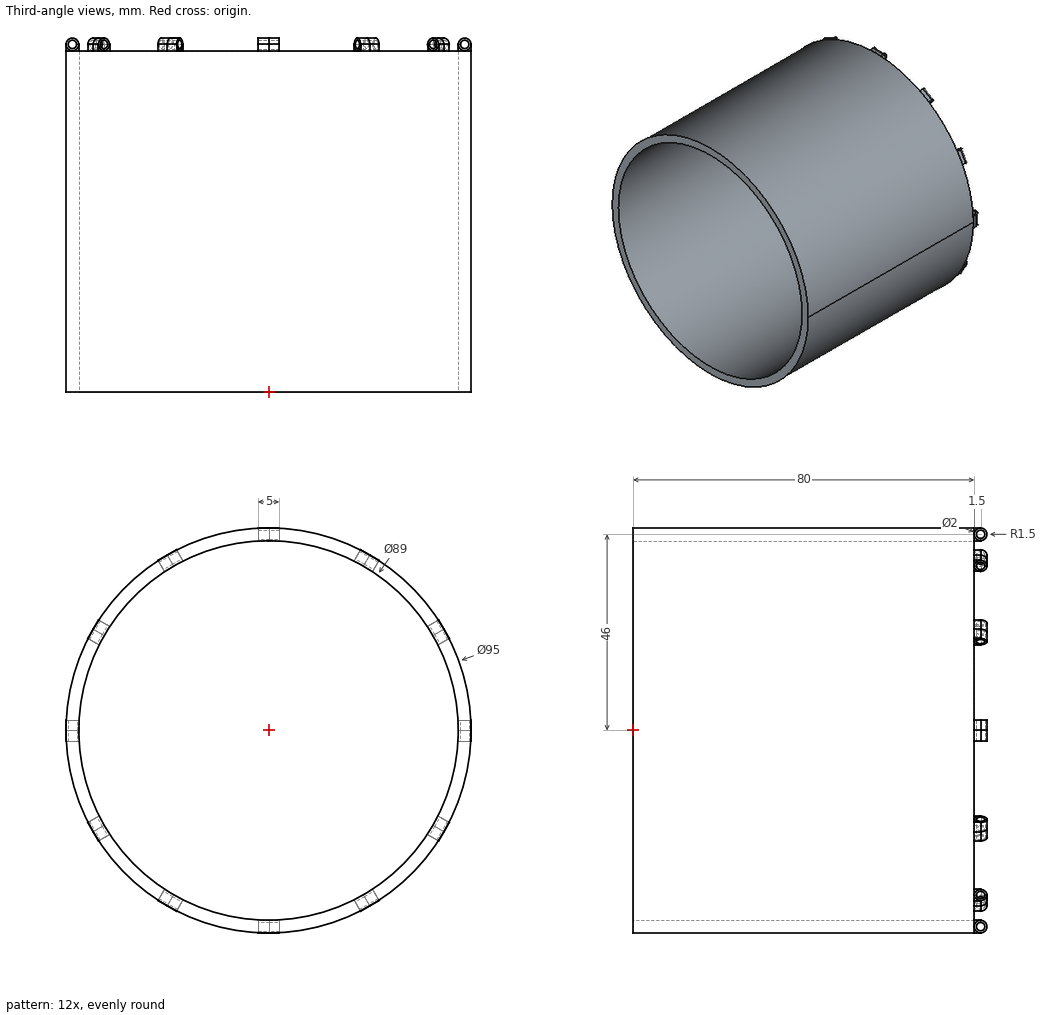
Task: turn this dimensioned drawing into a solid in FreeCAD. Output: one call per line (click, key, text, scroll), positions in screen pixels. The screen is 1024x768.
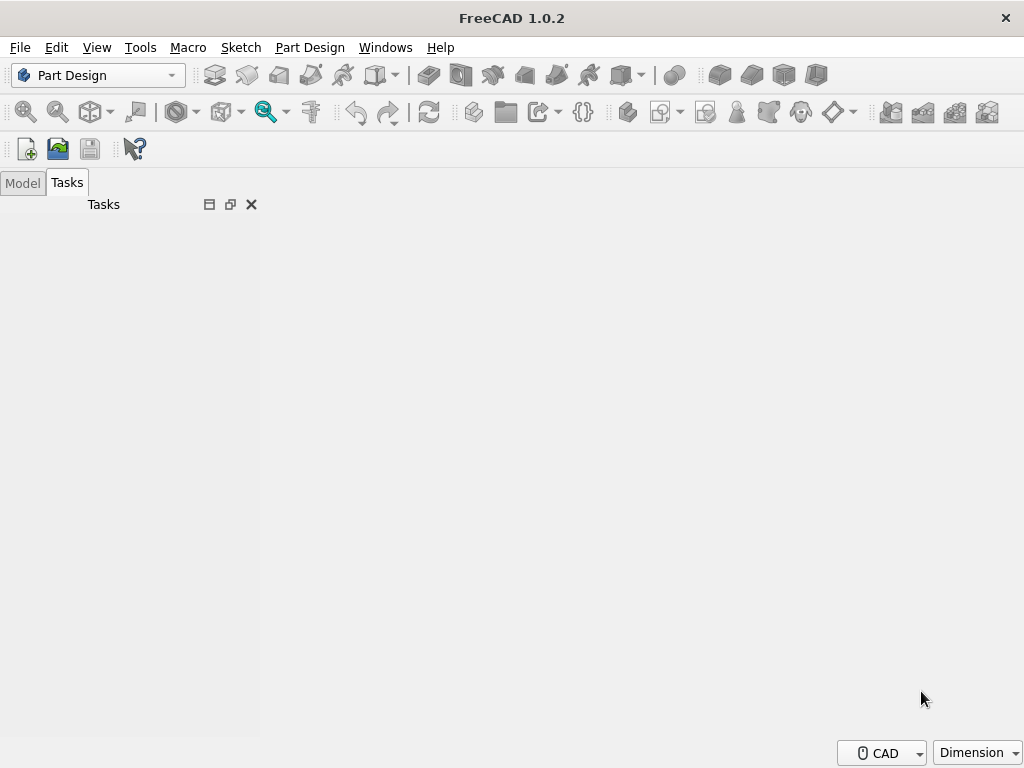
click(26, 150)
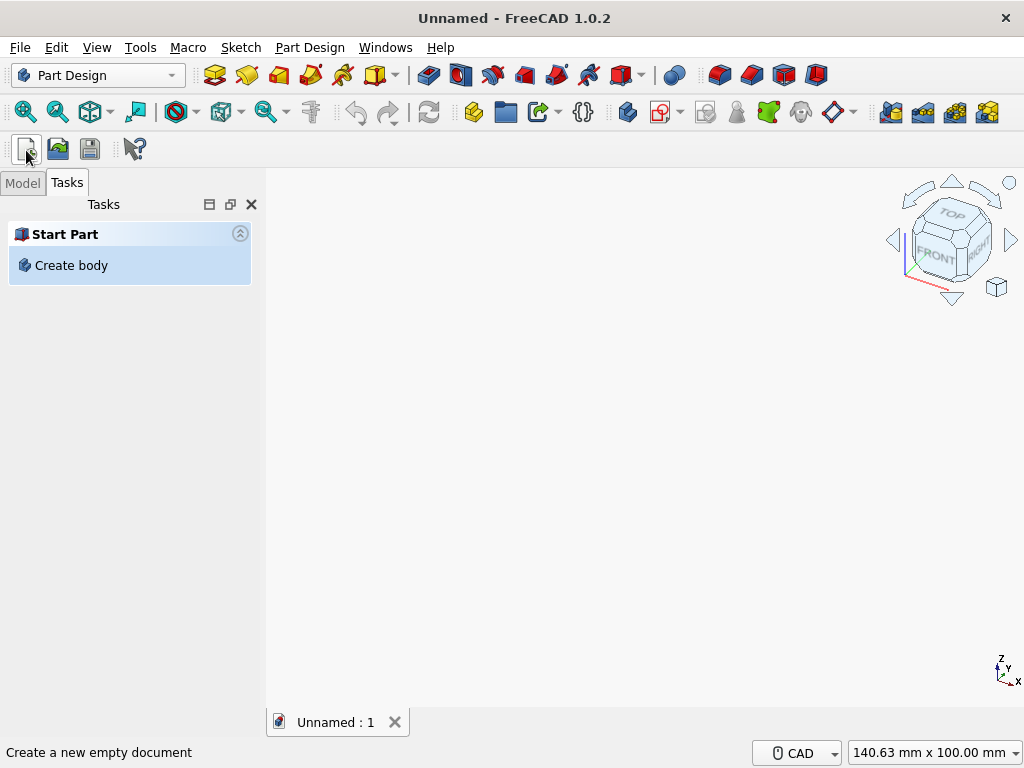
click(660, 112)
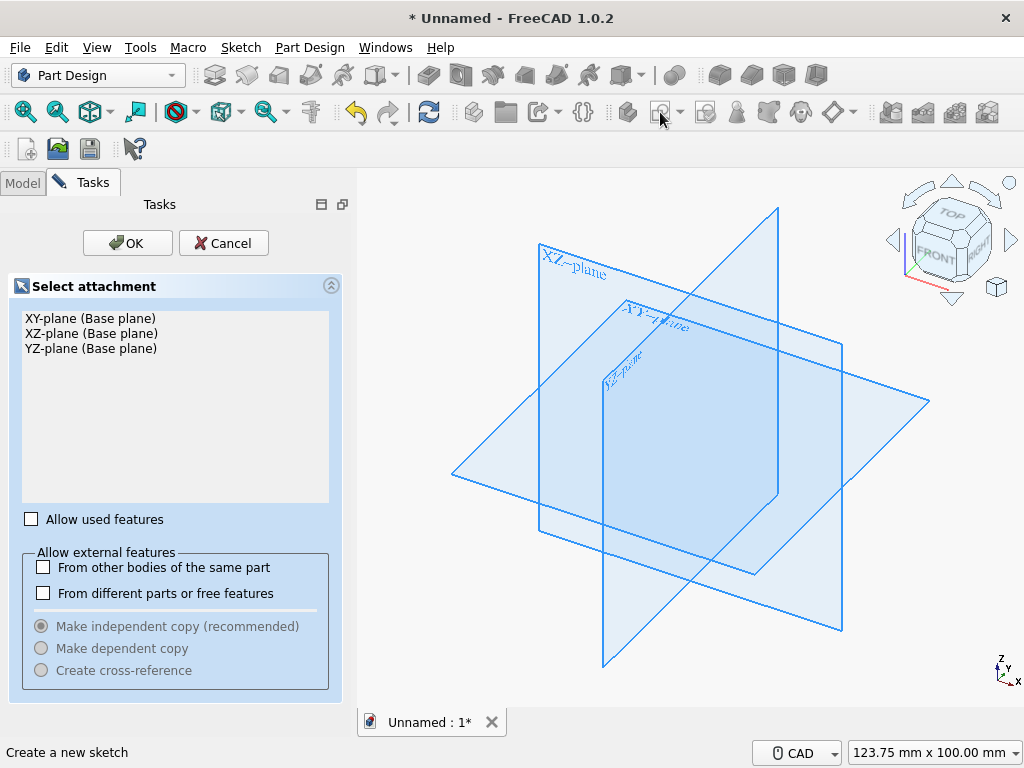
click(82, 334)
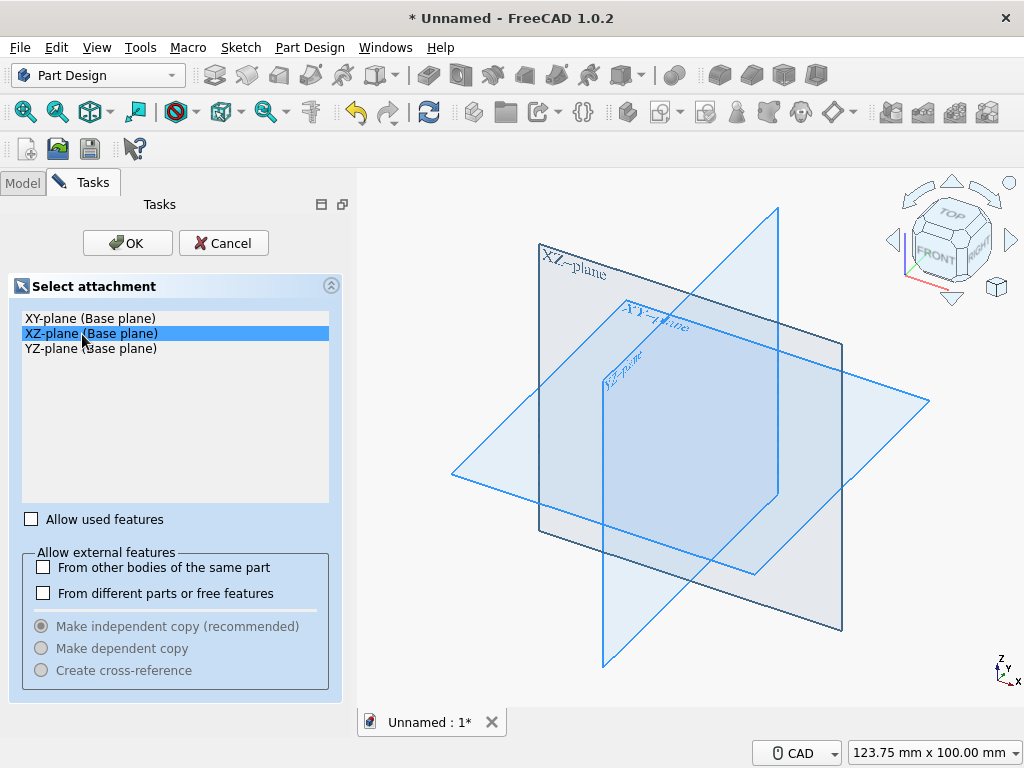
click(128, 243)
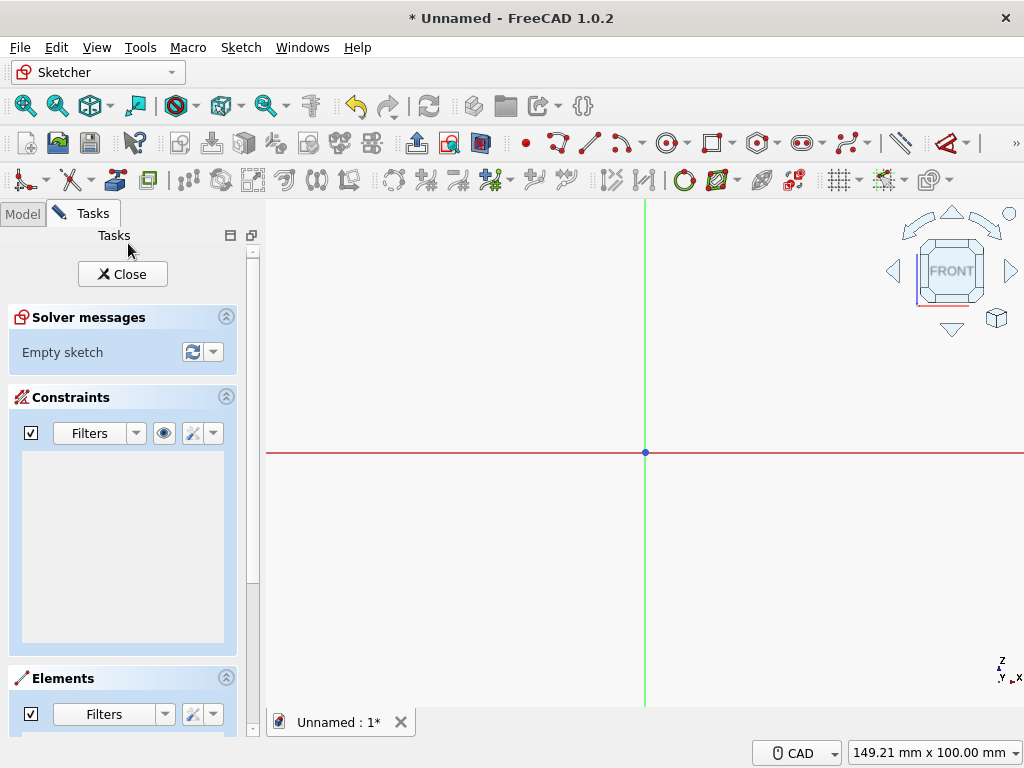
scroll(437, 453, down, 2)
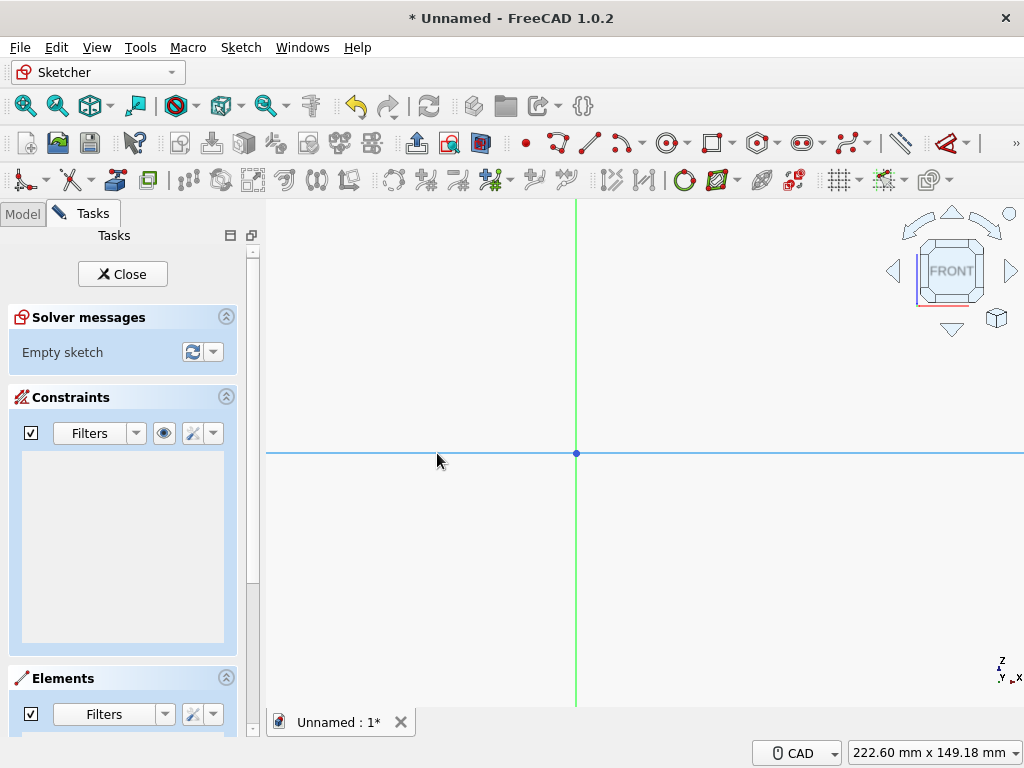
click(668, 144)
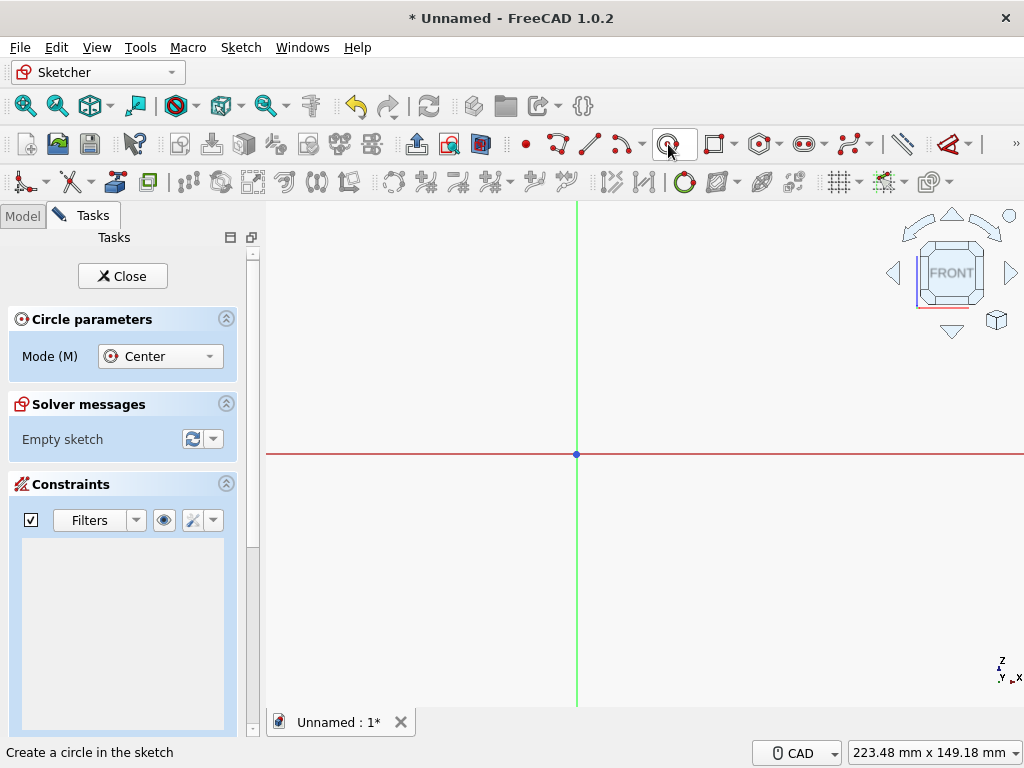
click(577, 454)
click(691, 340)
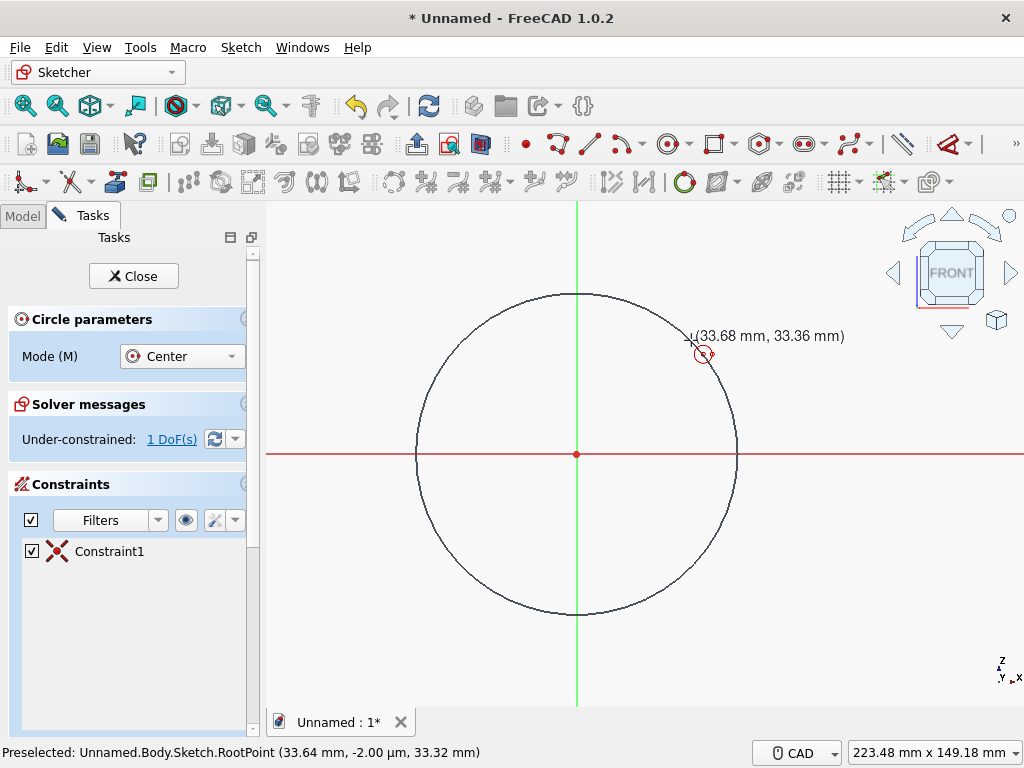
click(577, 454)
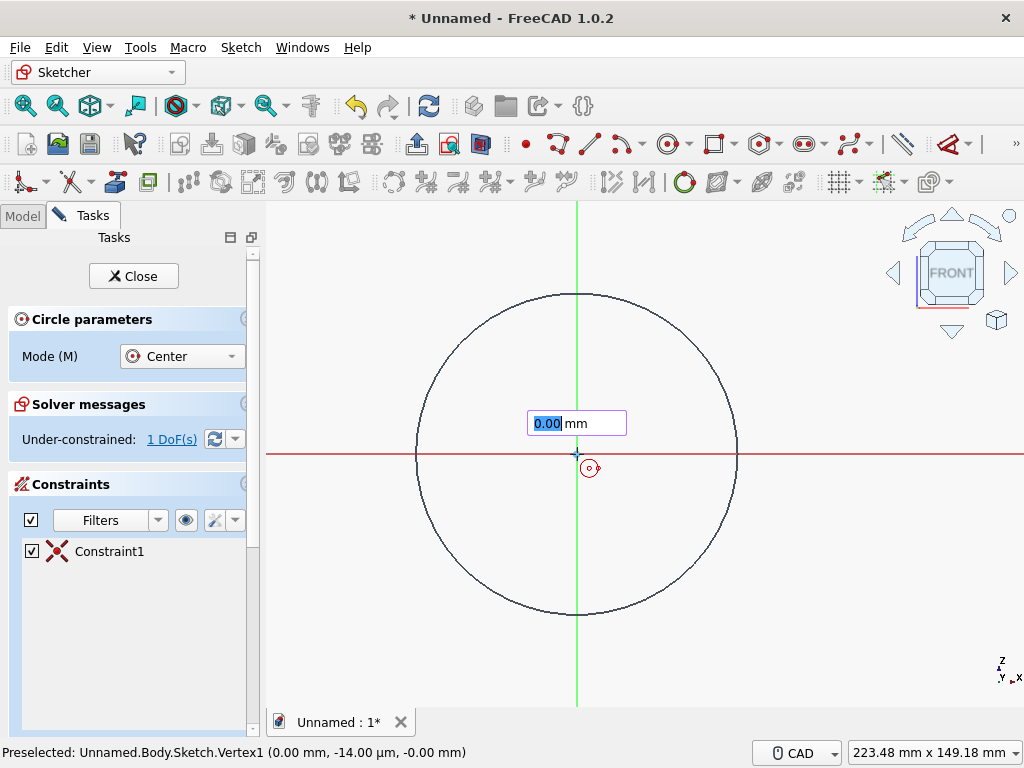
scroll(525, 596, up, 3)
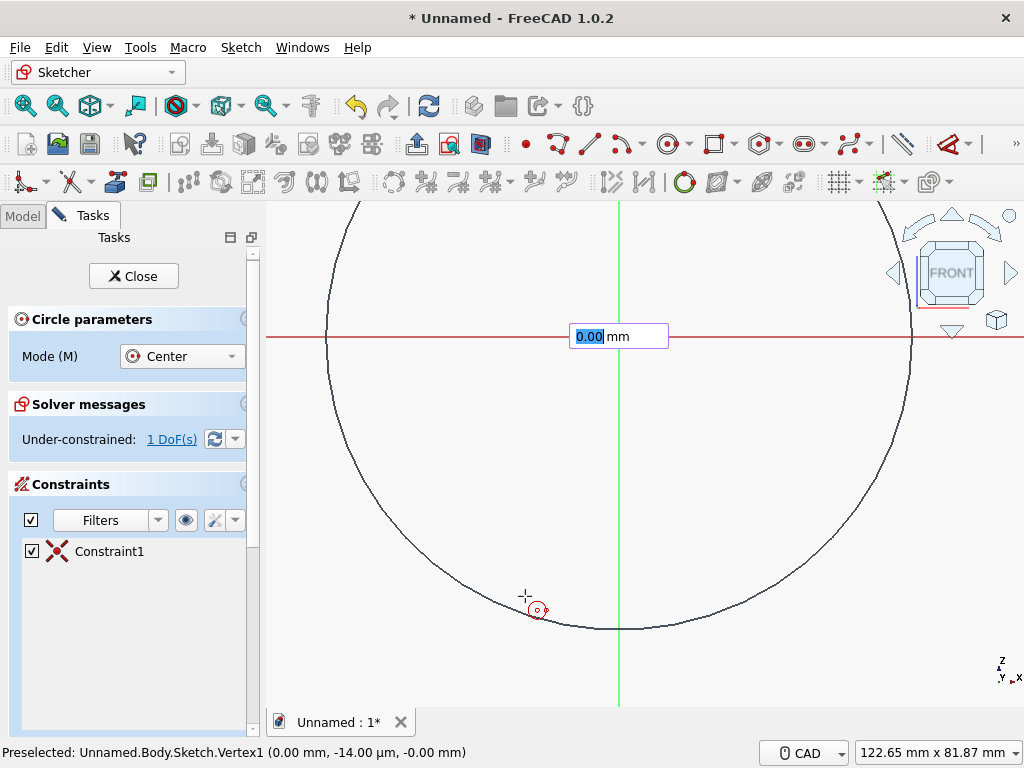
click(525, 595)
key(Escape)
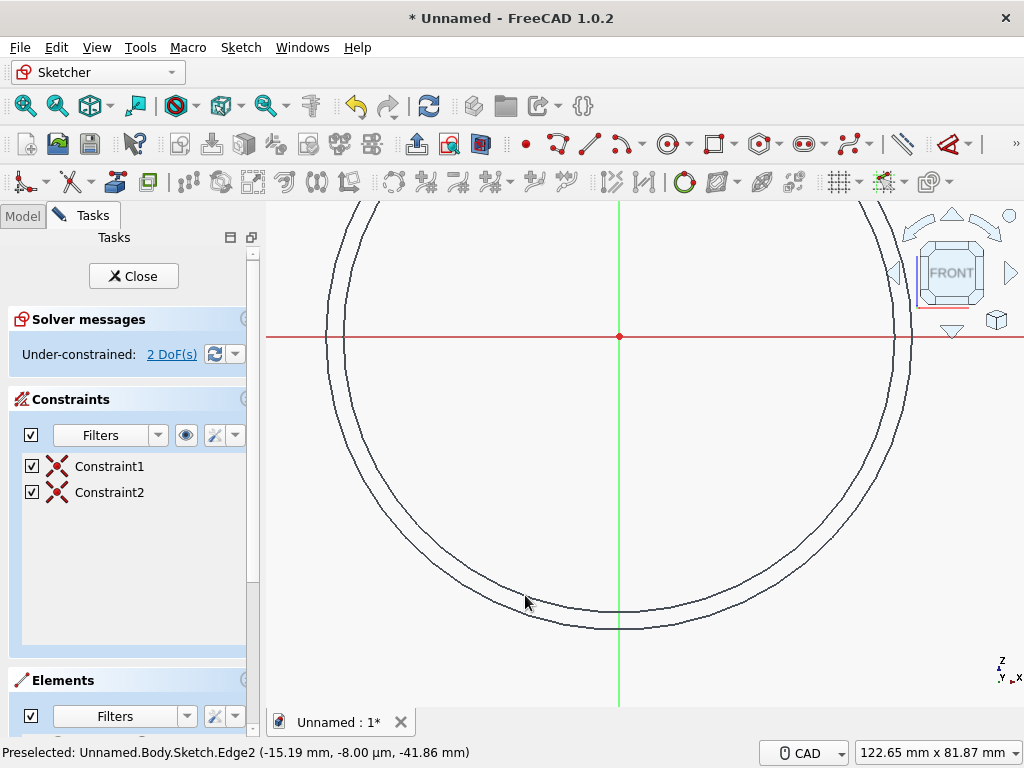
click(948, 144)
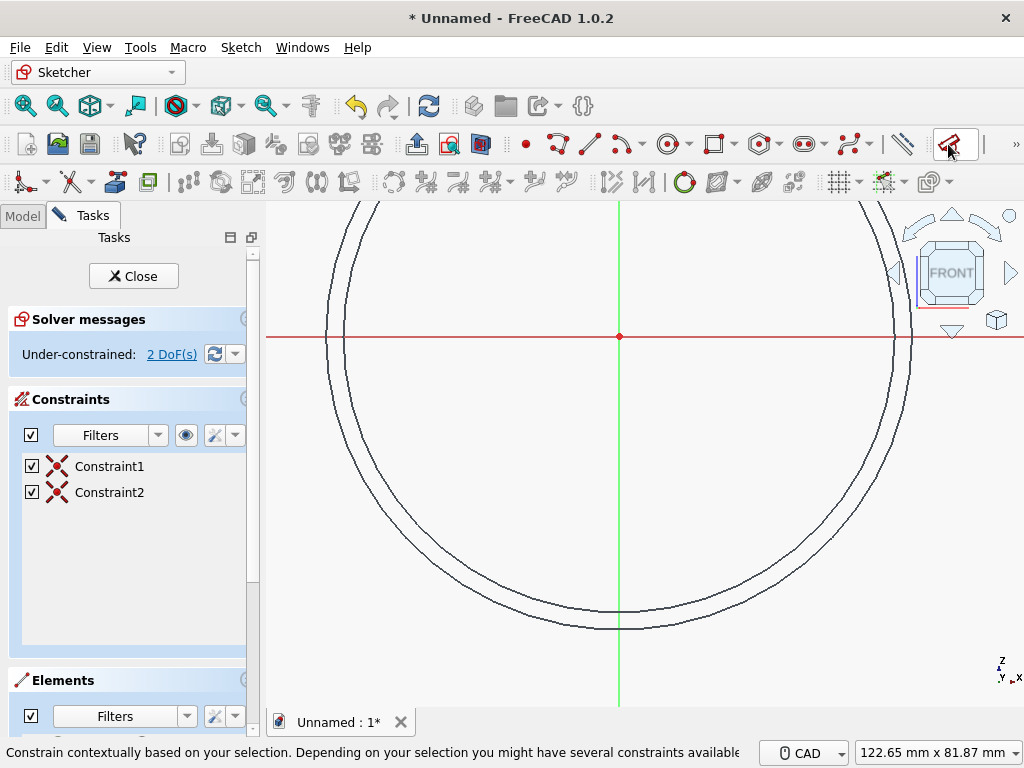
click(413, 545)
click(390, 568)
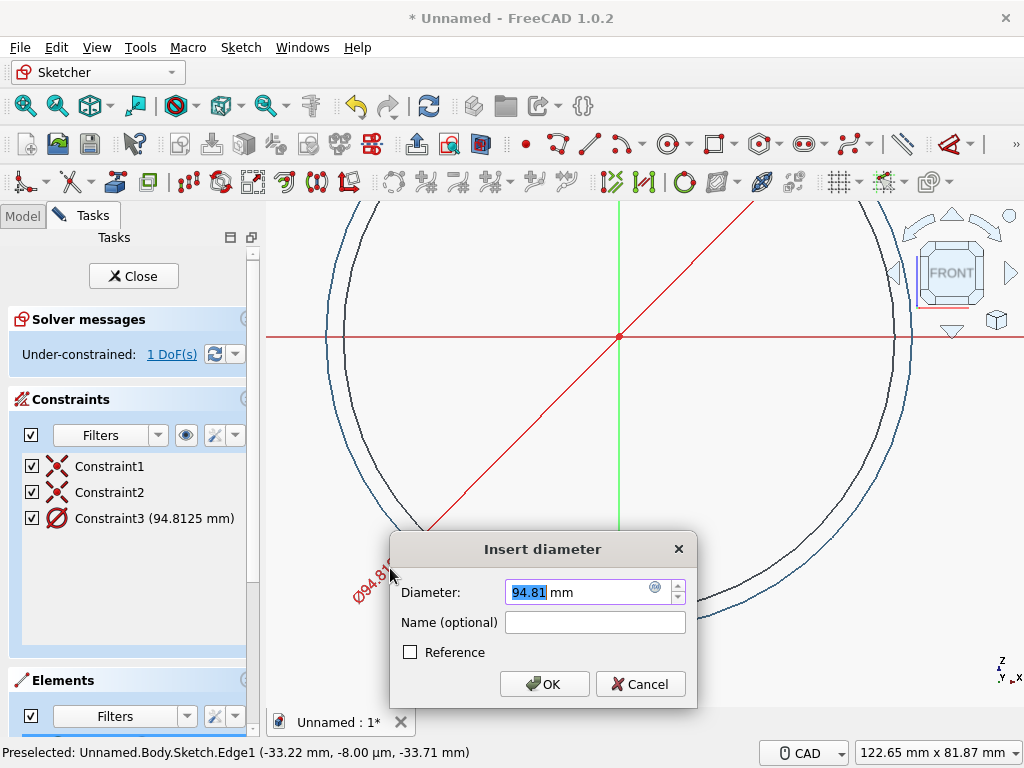
text(95)
key(Return)